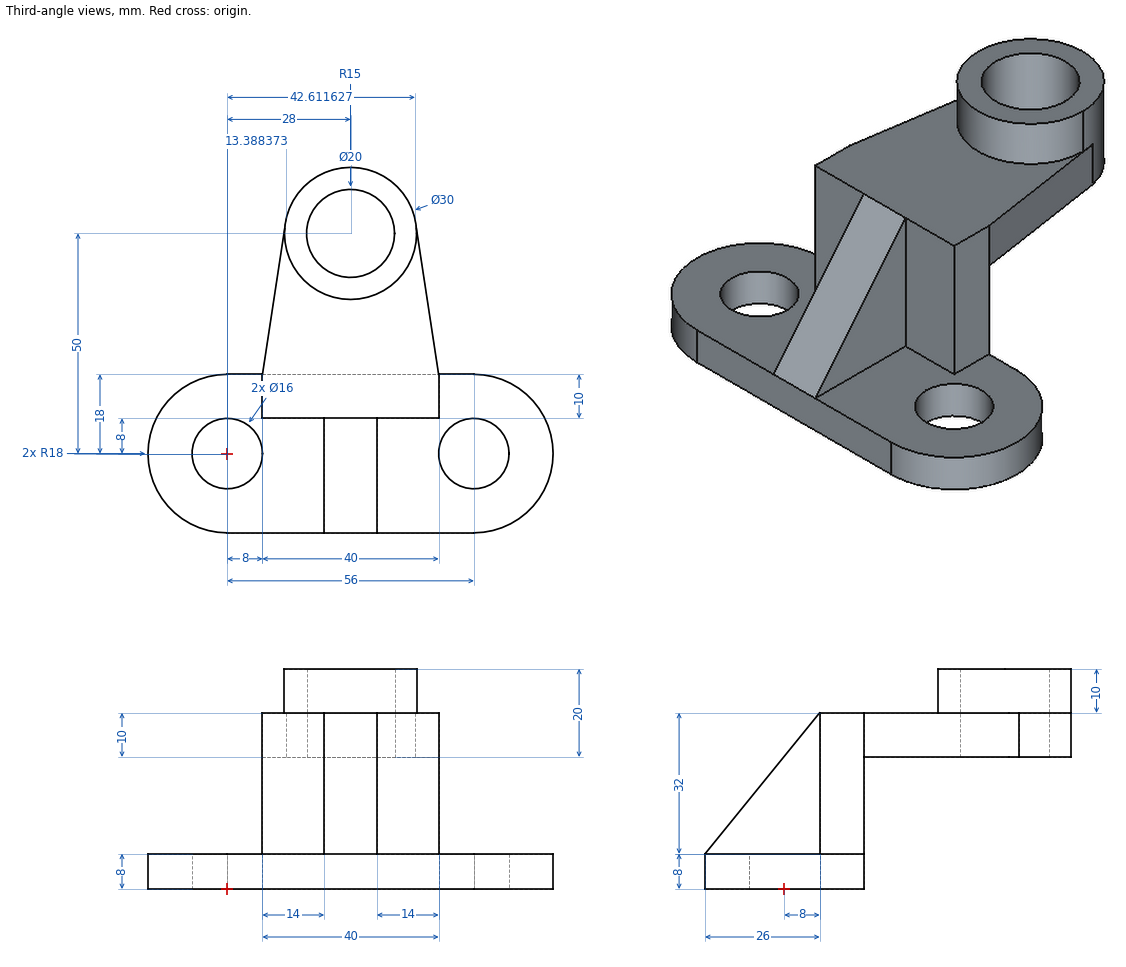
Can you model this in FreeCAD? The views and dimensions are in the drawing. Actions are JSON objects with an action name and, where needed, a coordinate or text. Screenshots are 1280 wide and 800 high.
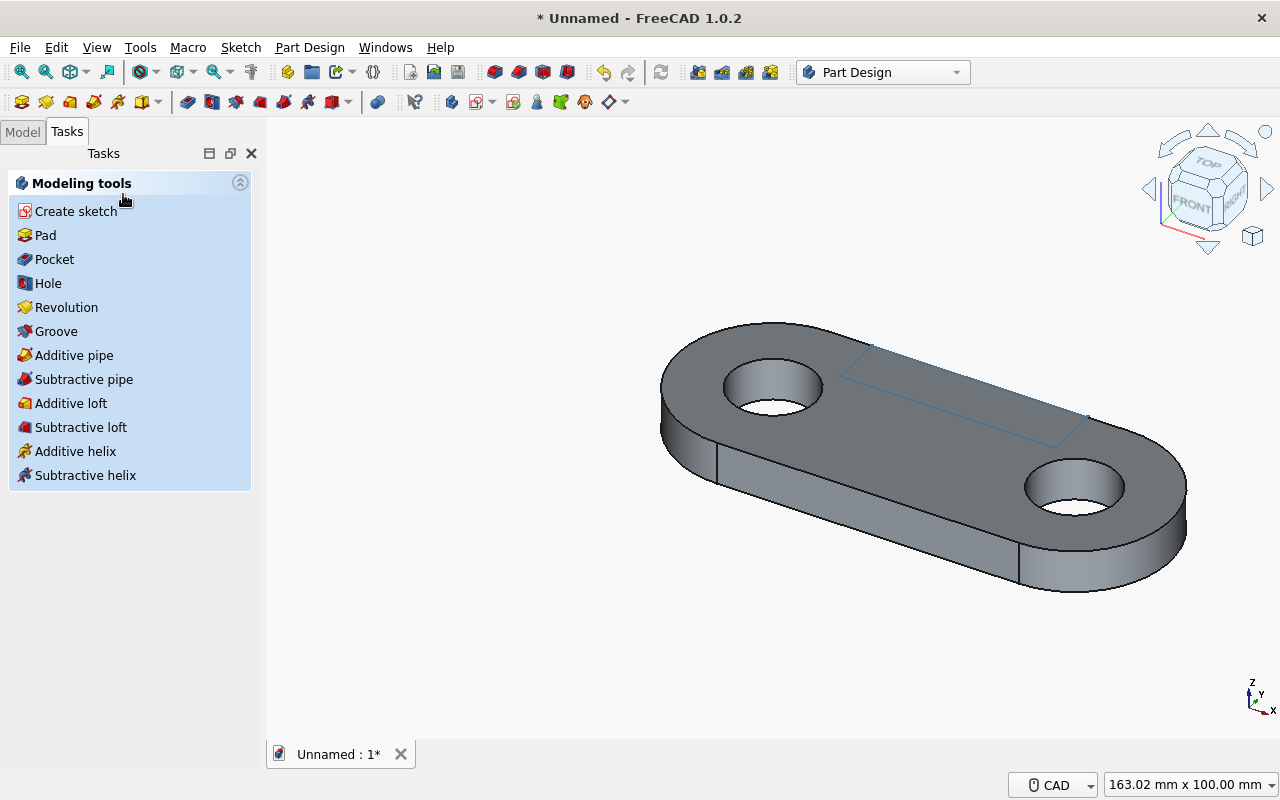
{"action": "left_click", "coordinate": [22, 102]}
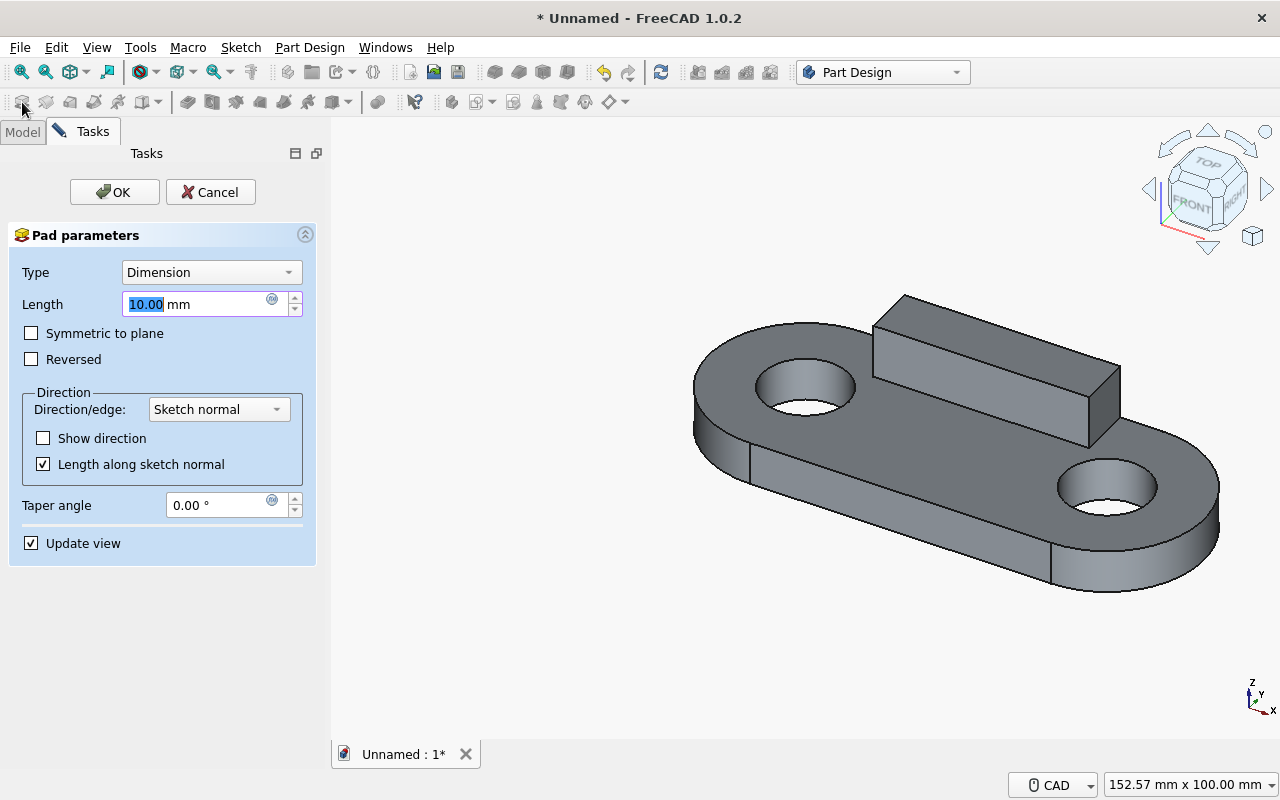
{"action": "type", "text": "32"}
{"action": "key", "text": "Tab"}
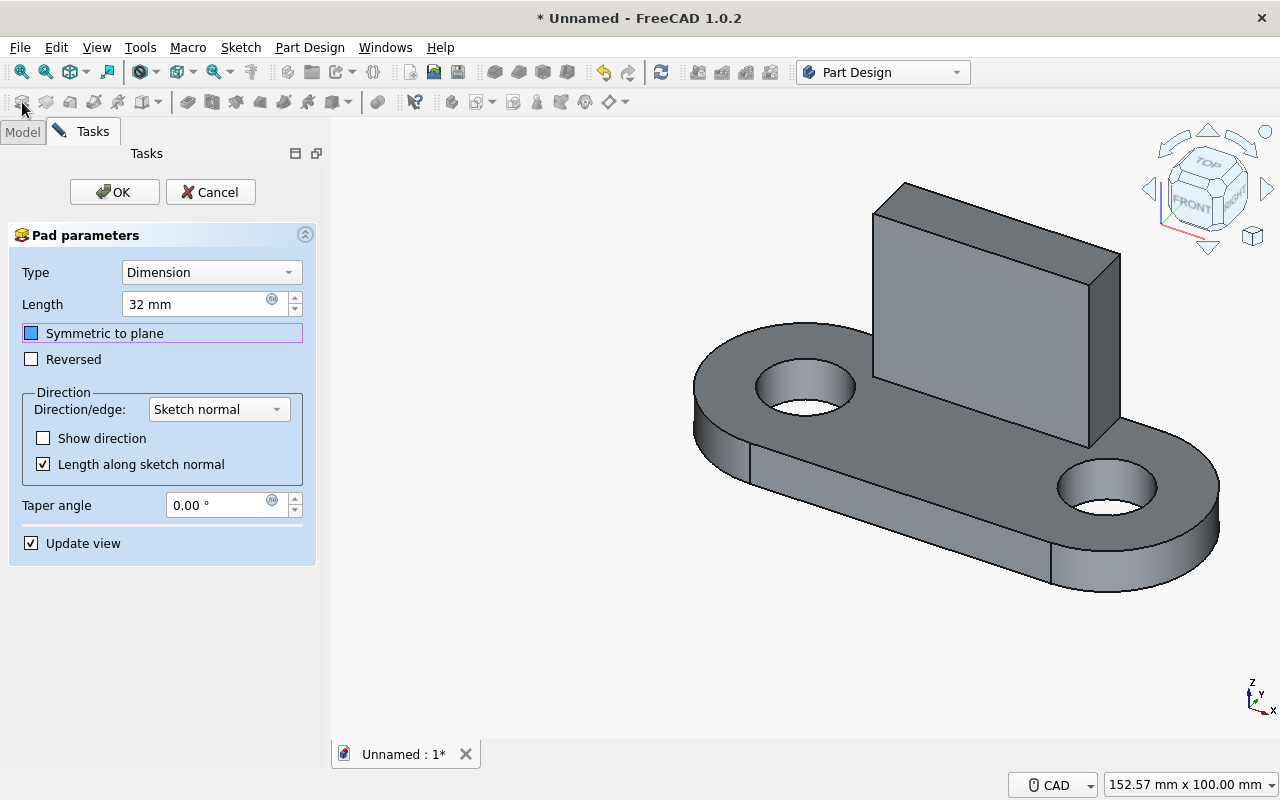
{"action": "left_click", "coordinate": [115, 192]}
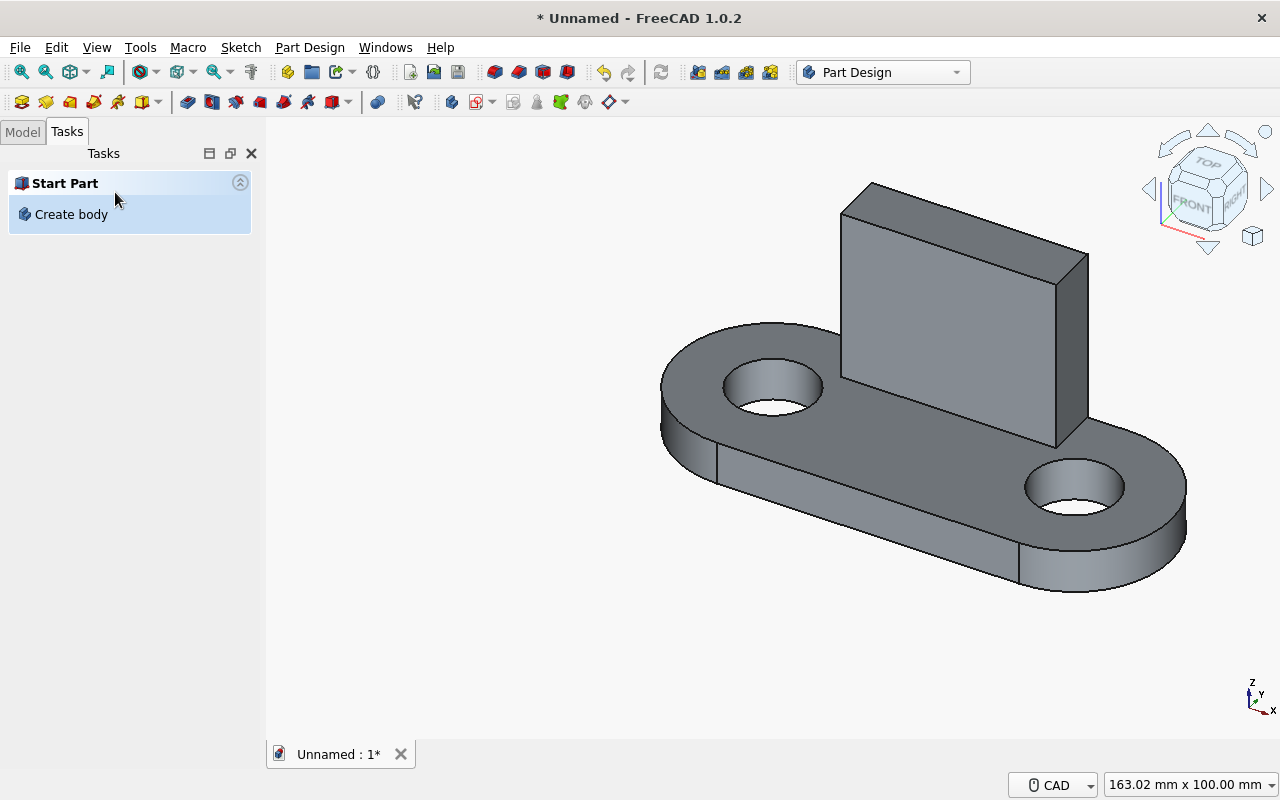
{"action": "left_click", "coordinate": [1026, 253]}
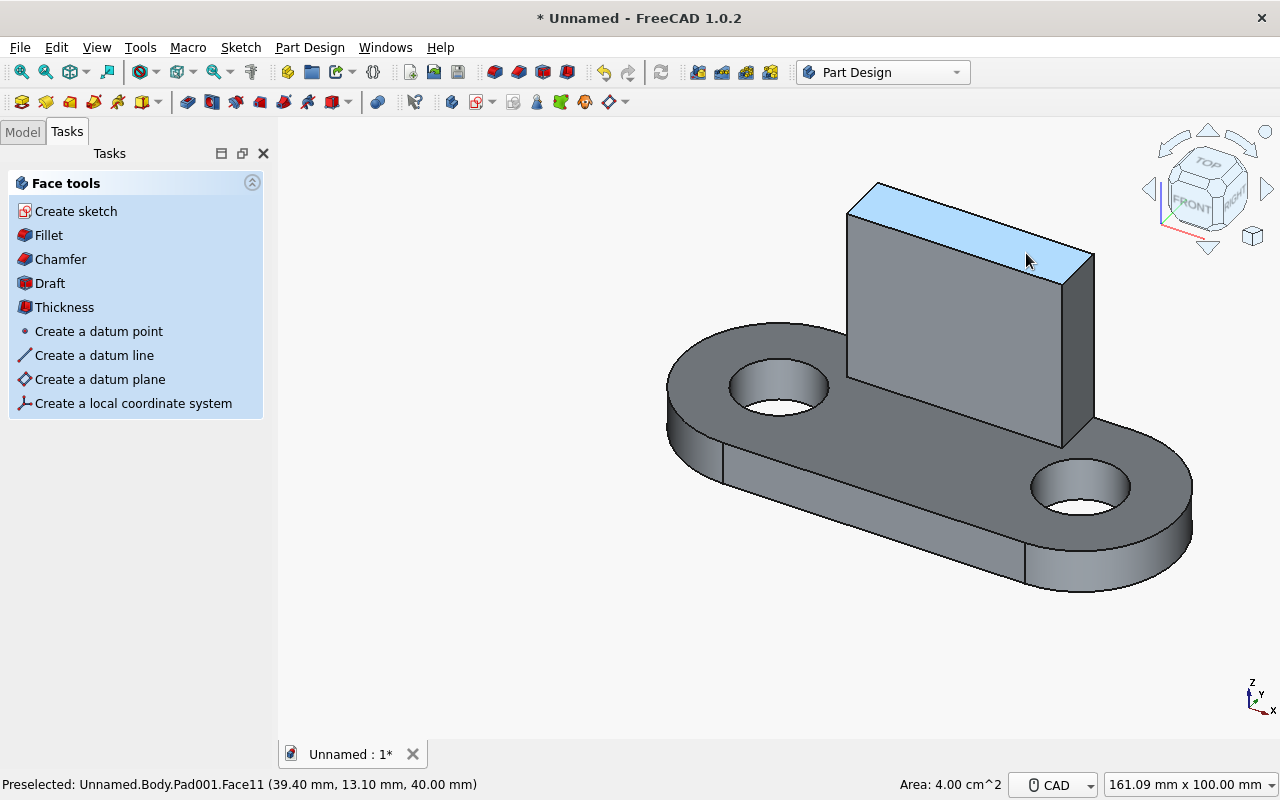
{"action": "left_click", "coordinate": [476, 102]}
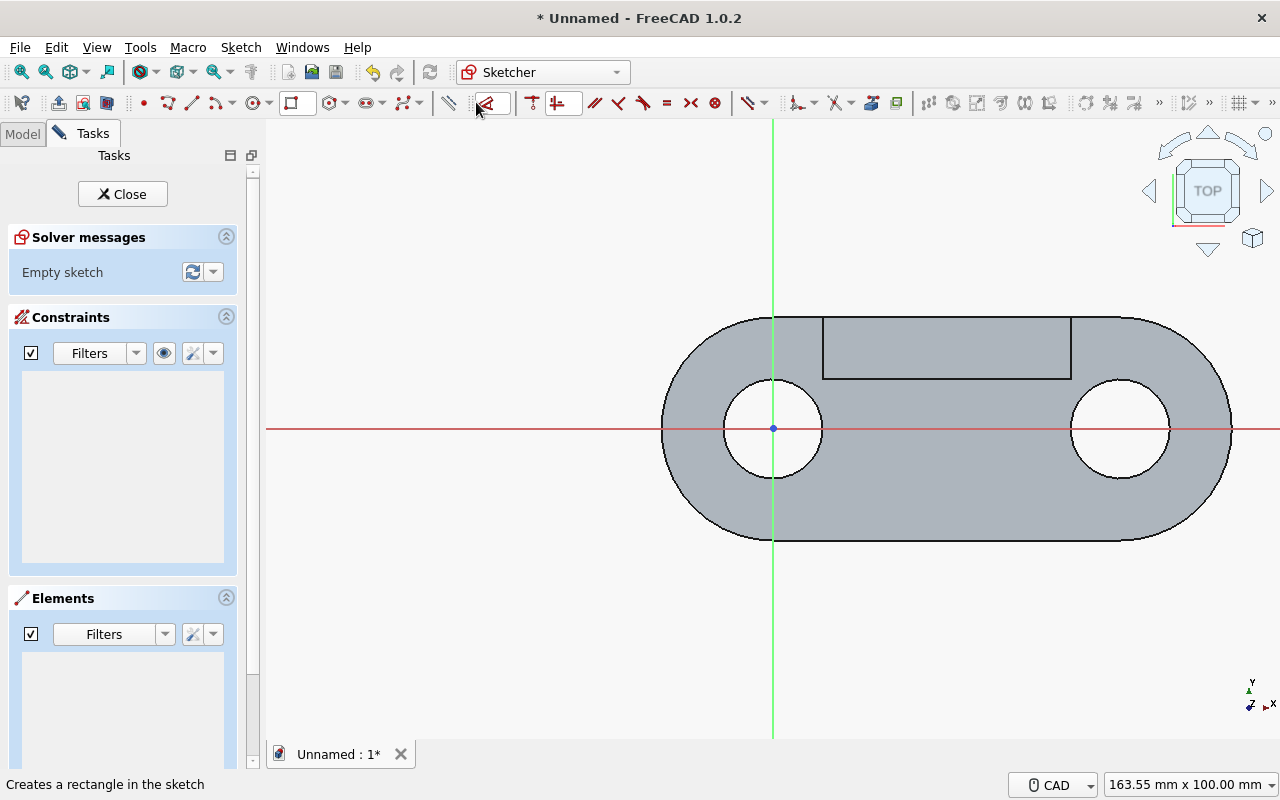
{"action": "scroll", "coordinate": [294, 711], "scroll_direction": "down", "scroll_amount": 2}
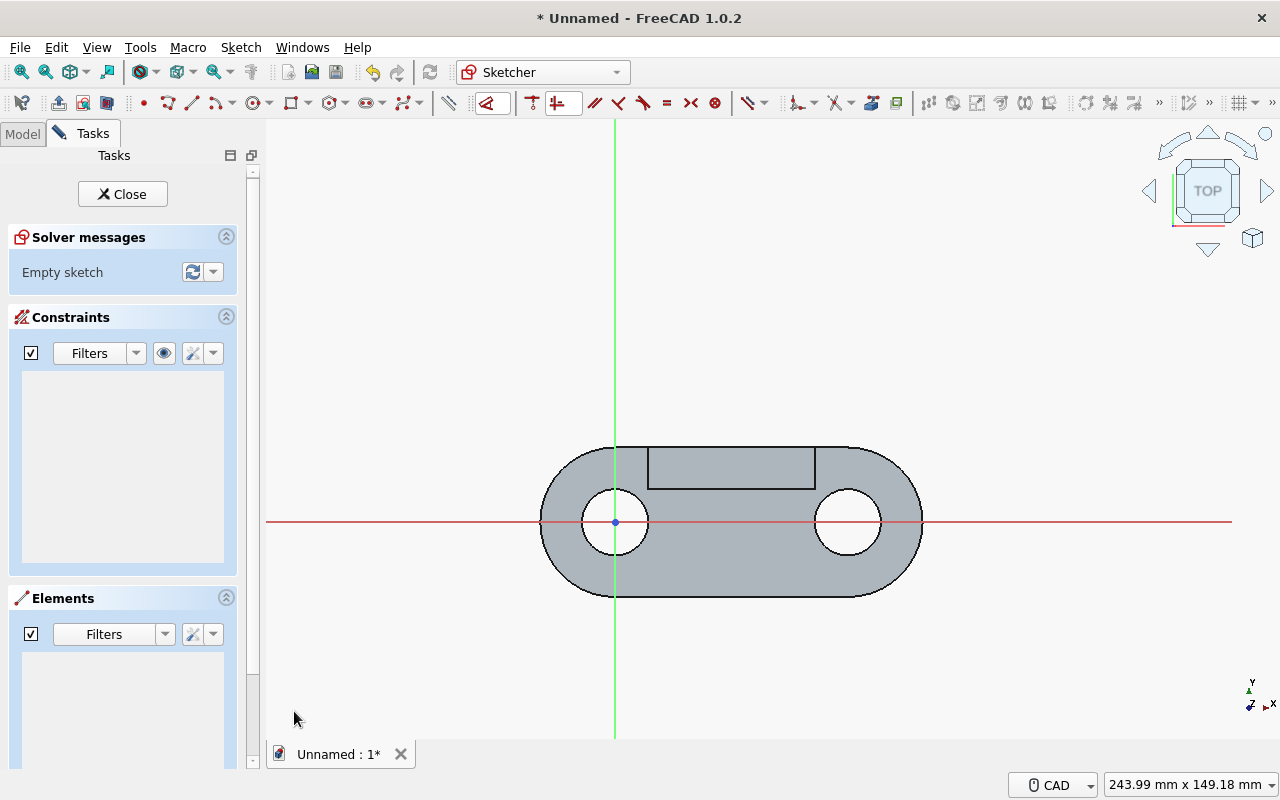
{"action": "scroll", "coordinate": [736, 302], "scroll_direction": "up", "scroll_amount": 2}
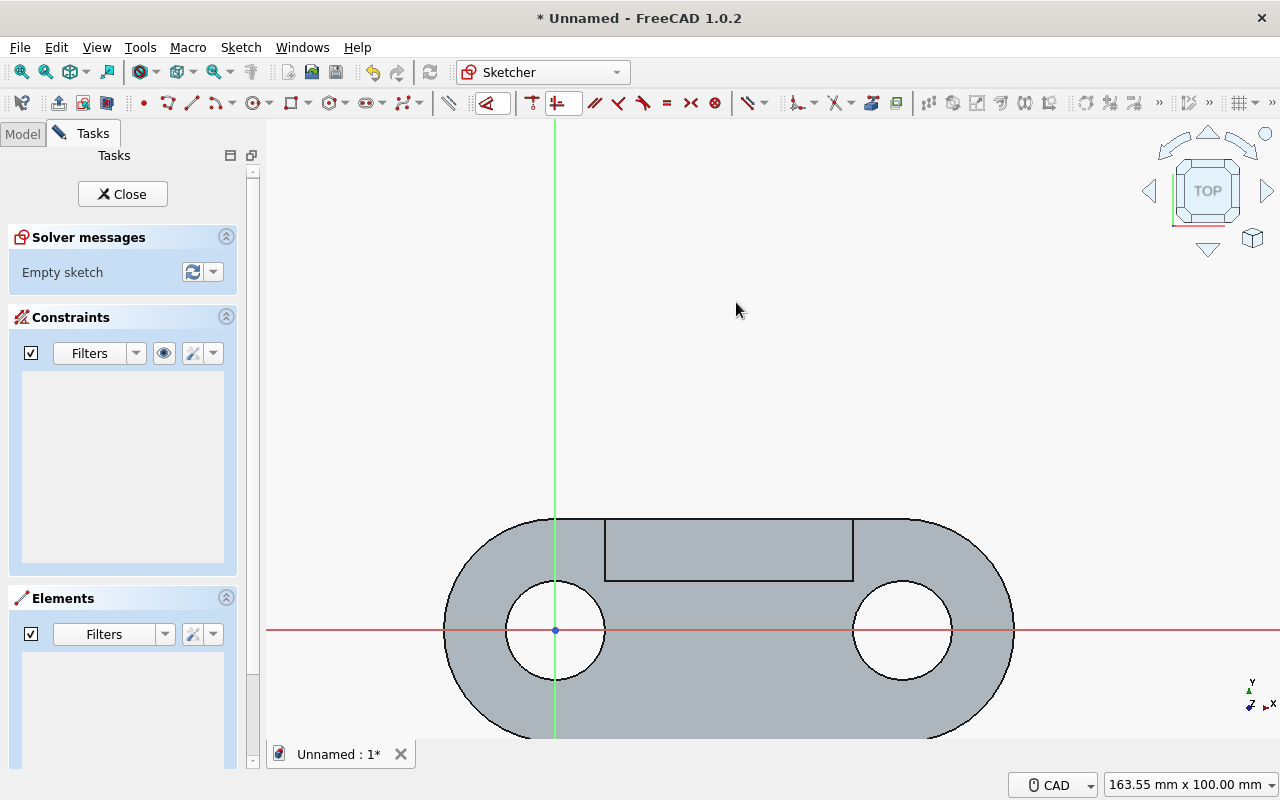
{"action": "left_click", "coordinate": [168, 104]}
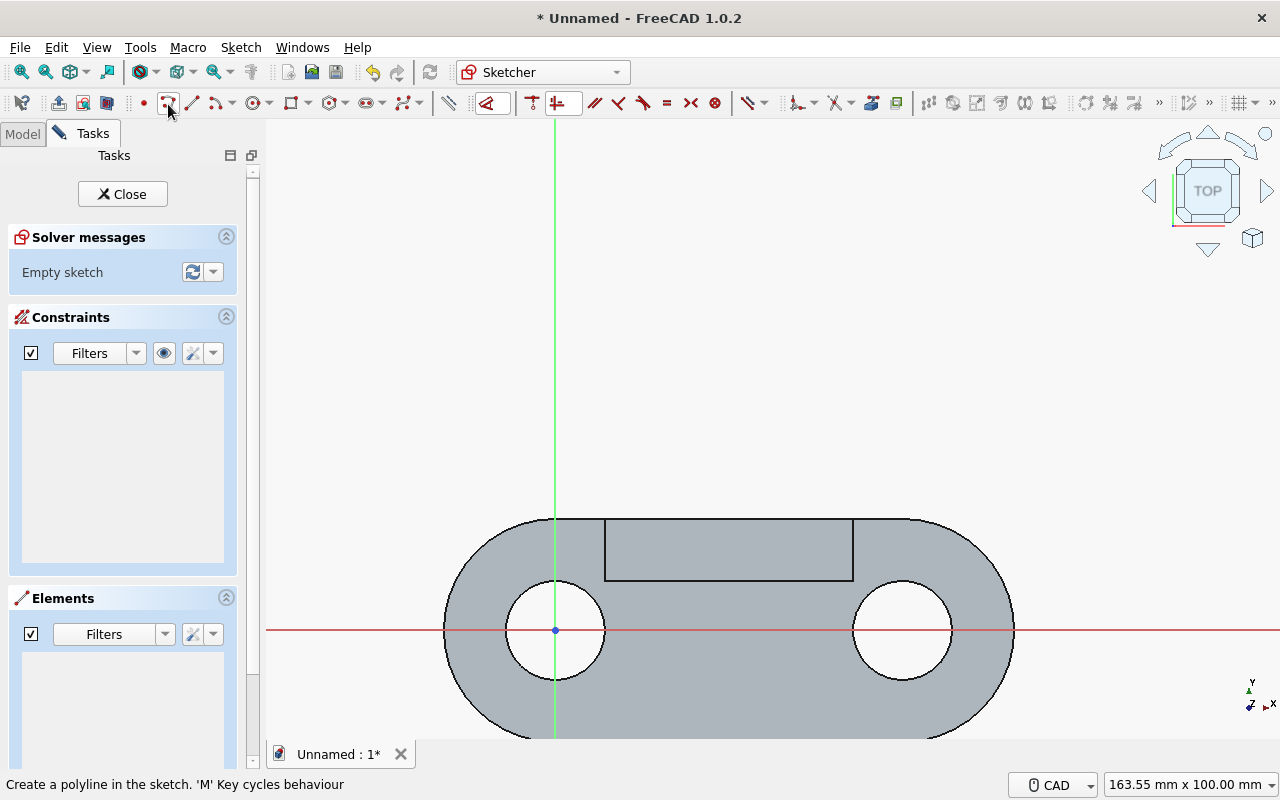
{"action": "left_click", "coordinate": [638, 299]}
{"action": "left_click", "coordinate": [605, 519]}
{"action": "left_click", "coordinate": [853, 519]}
{"action": "left_click", "coordinate": [820, 299]}
{"action": "right_click", "coordinate": [820, 299]}